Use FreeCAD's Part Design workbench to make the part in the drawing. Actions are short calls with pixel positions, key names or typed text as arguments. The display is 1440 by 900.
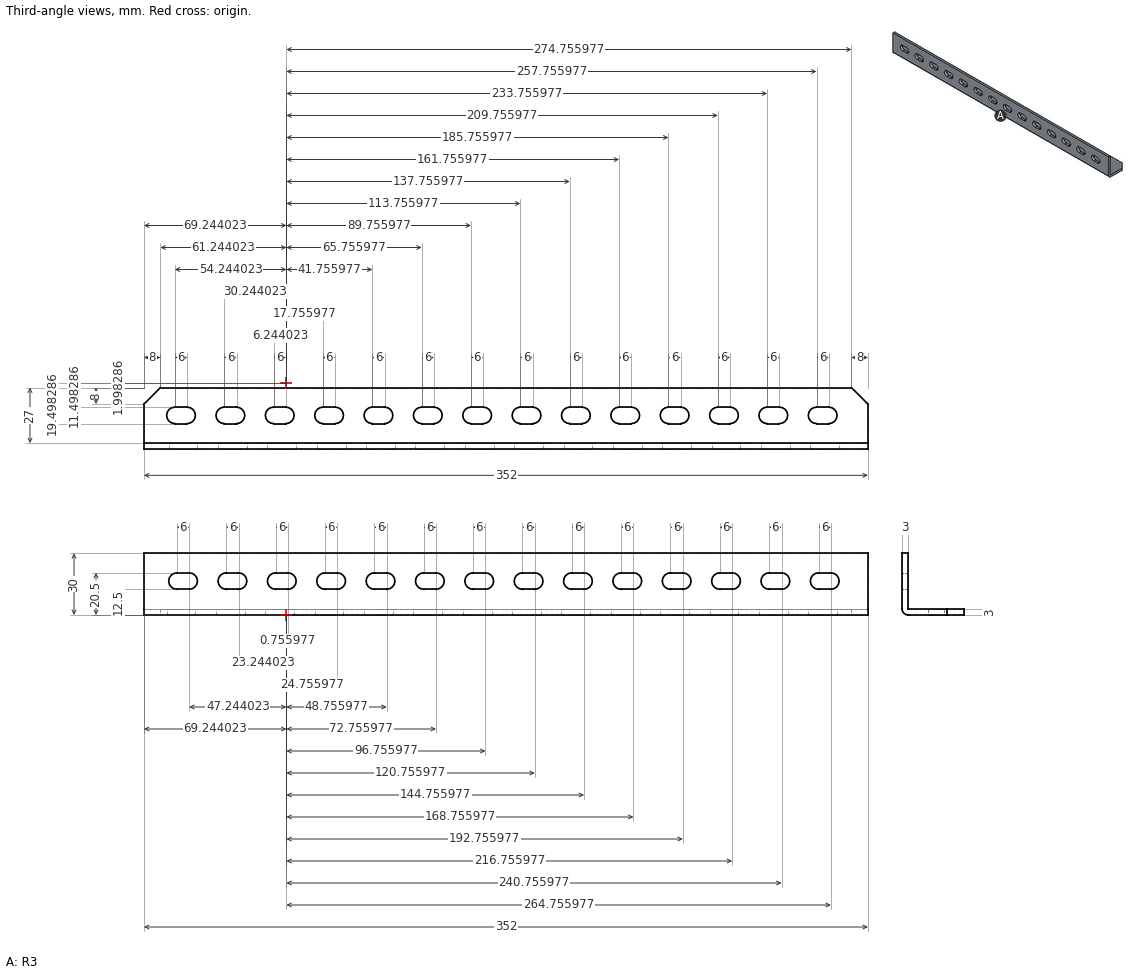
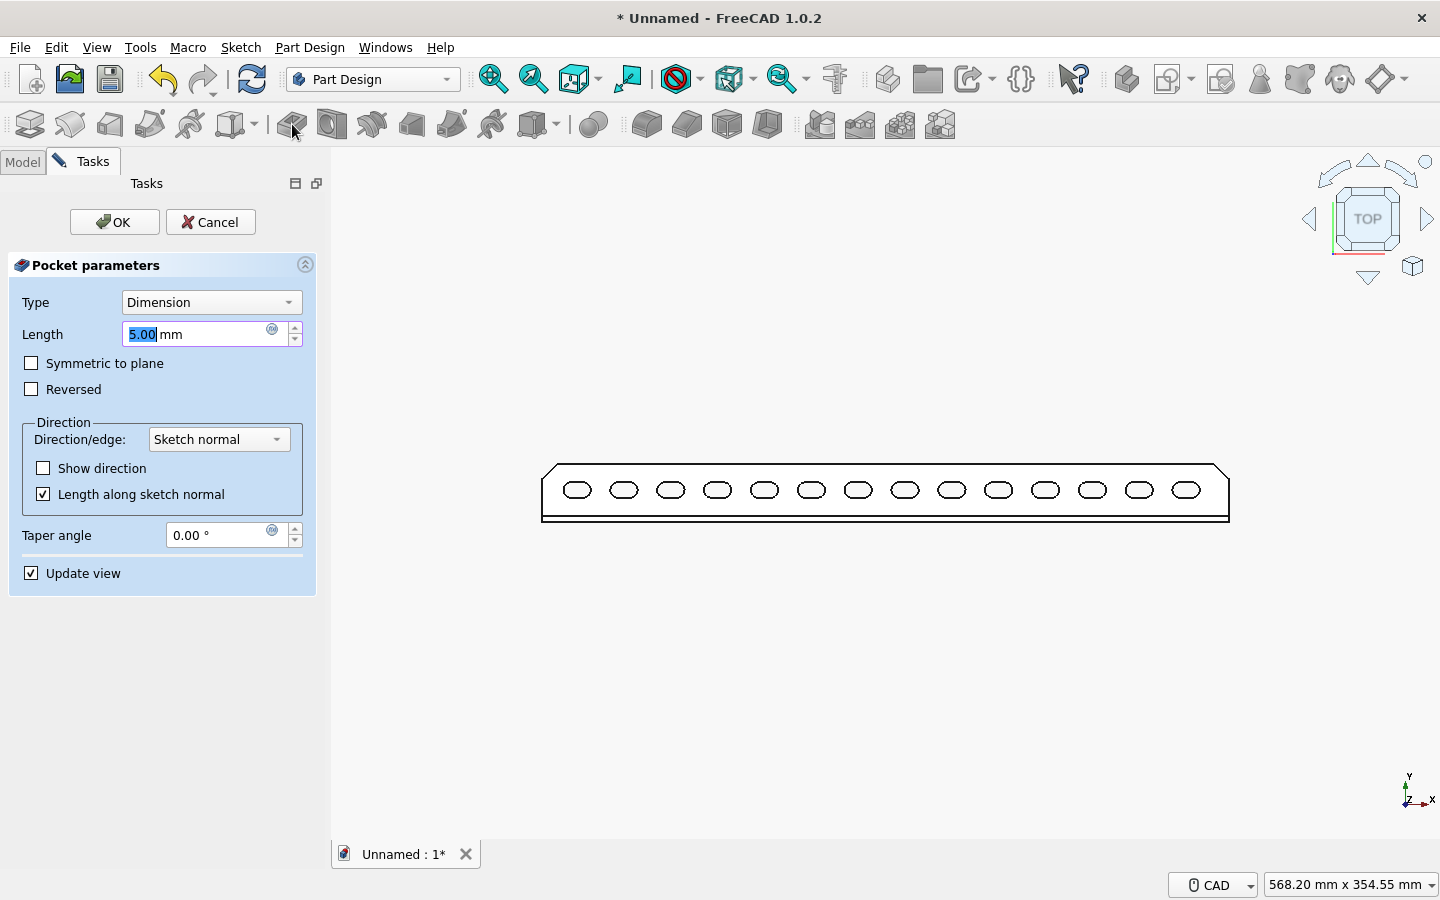
text(3)
key(Tab)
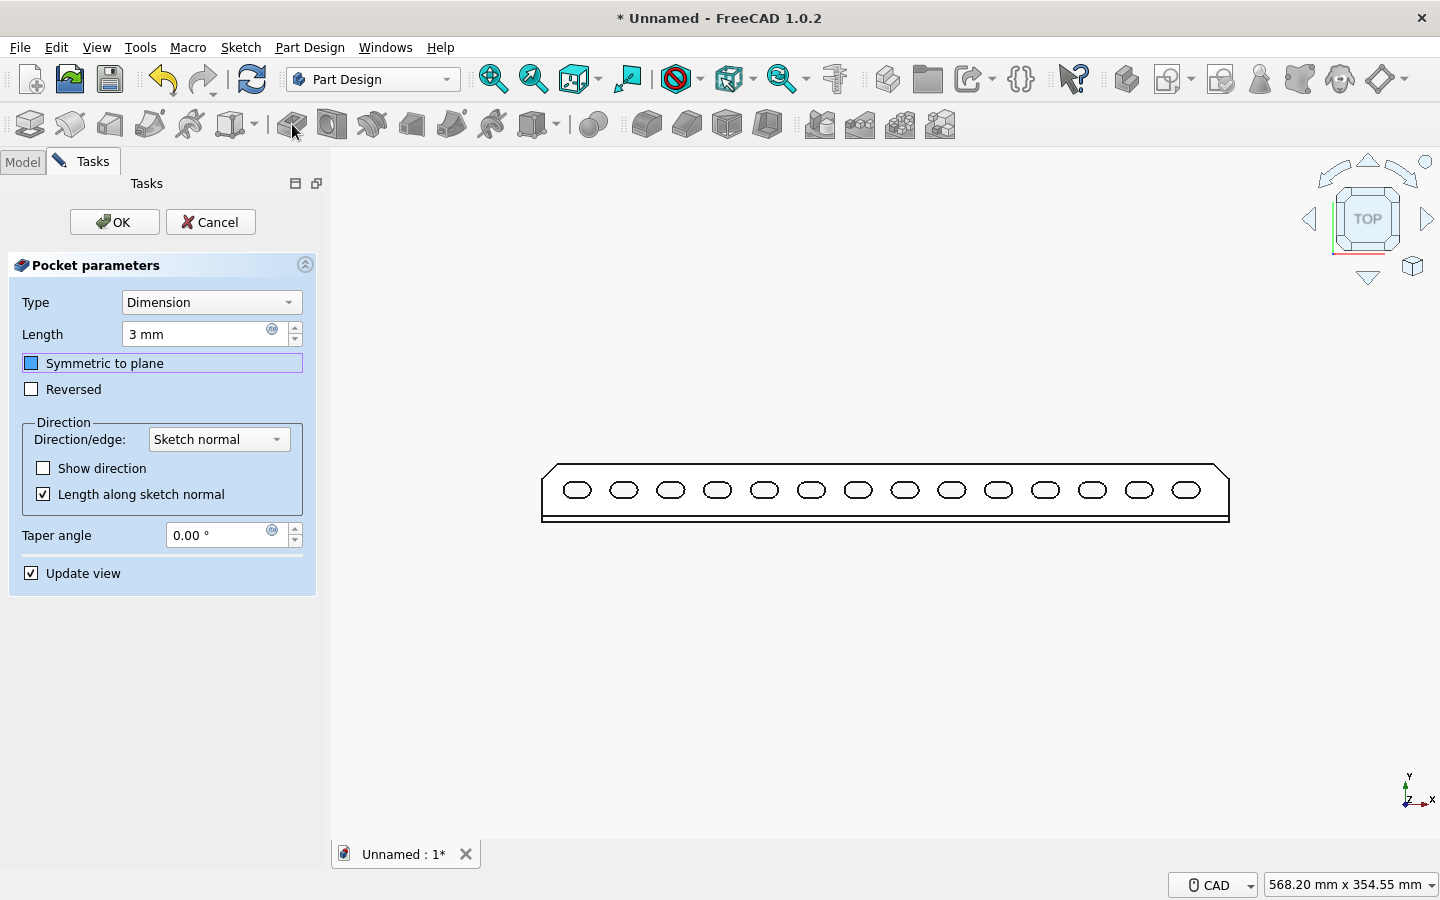
click(115, 222)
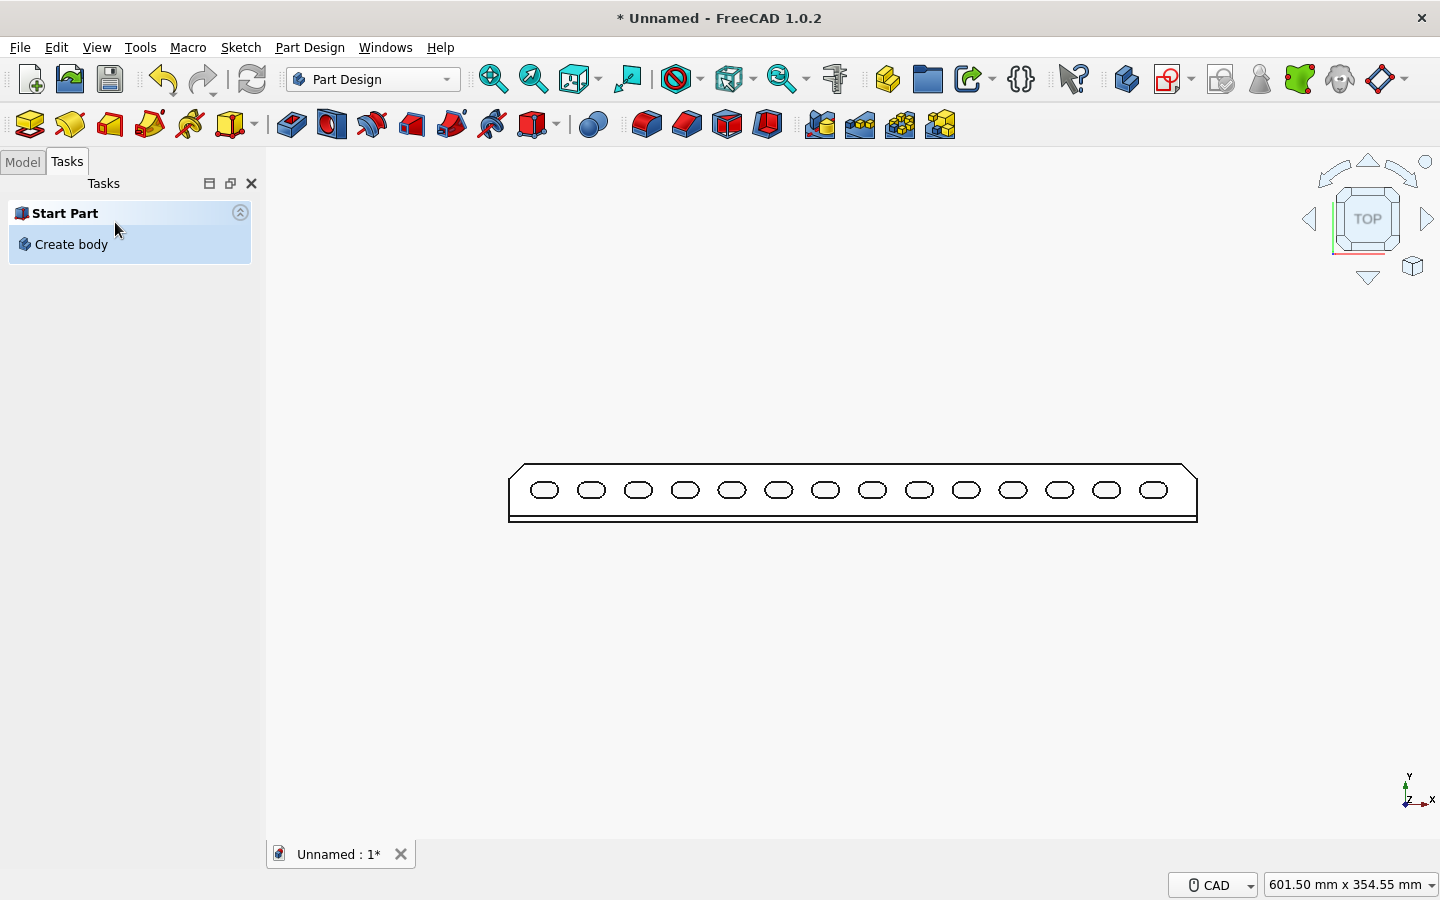
key(0)